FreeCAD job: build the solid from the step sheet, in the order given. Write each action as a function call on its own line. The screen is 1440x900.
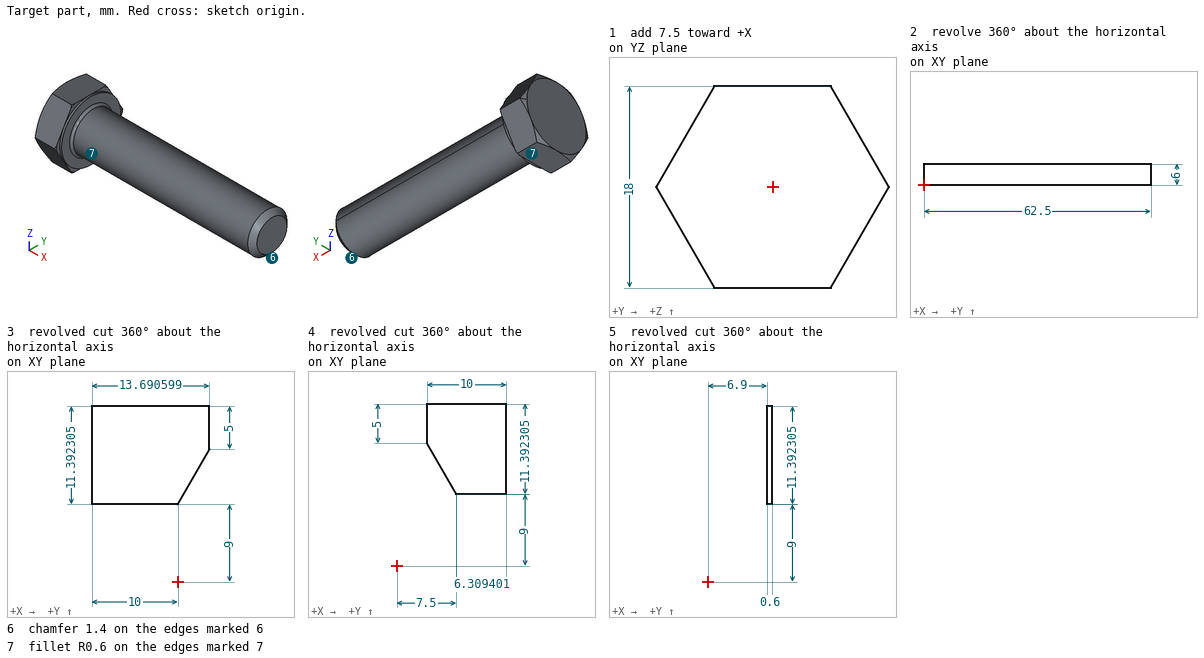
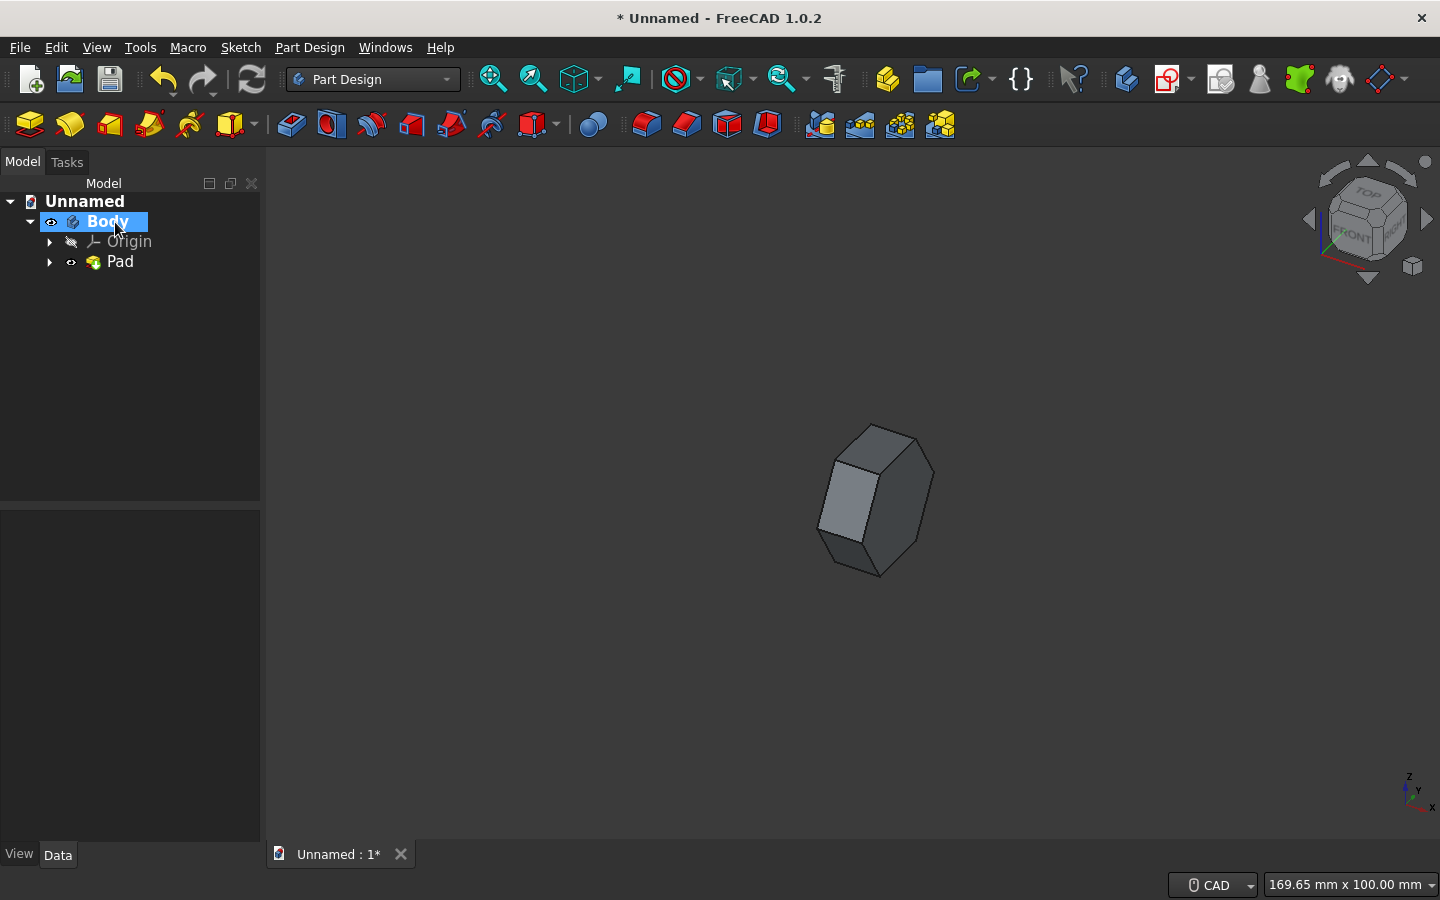
click(494, 80)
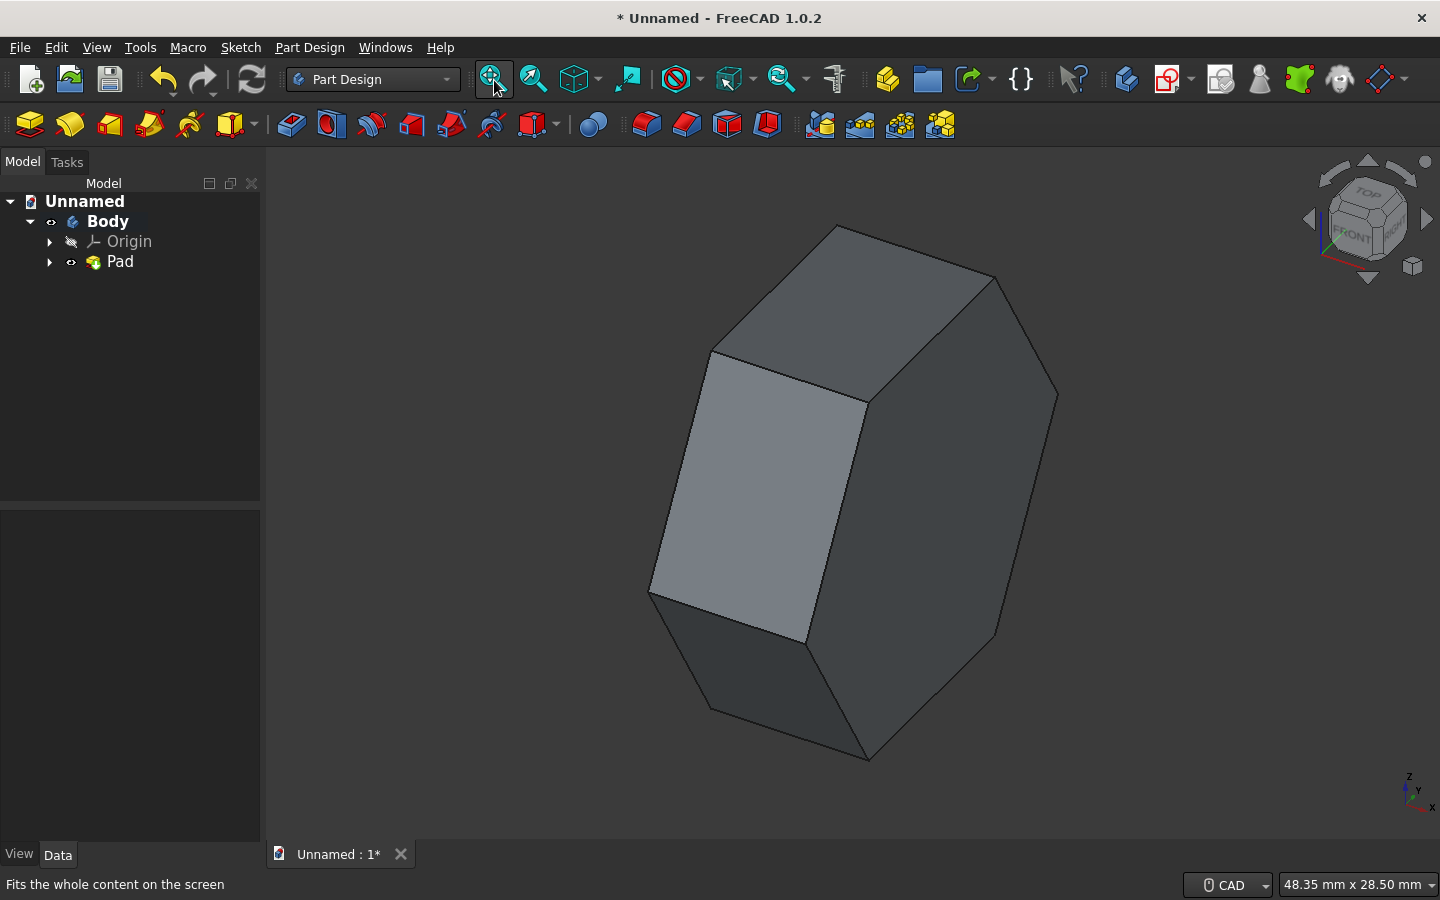
click(1168, 80)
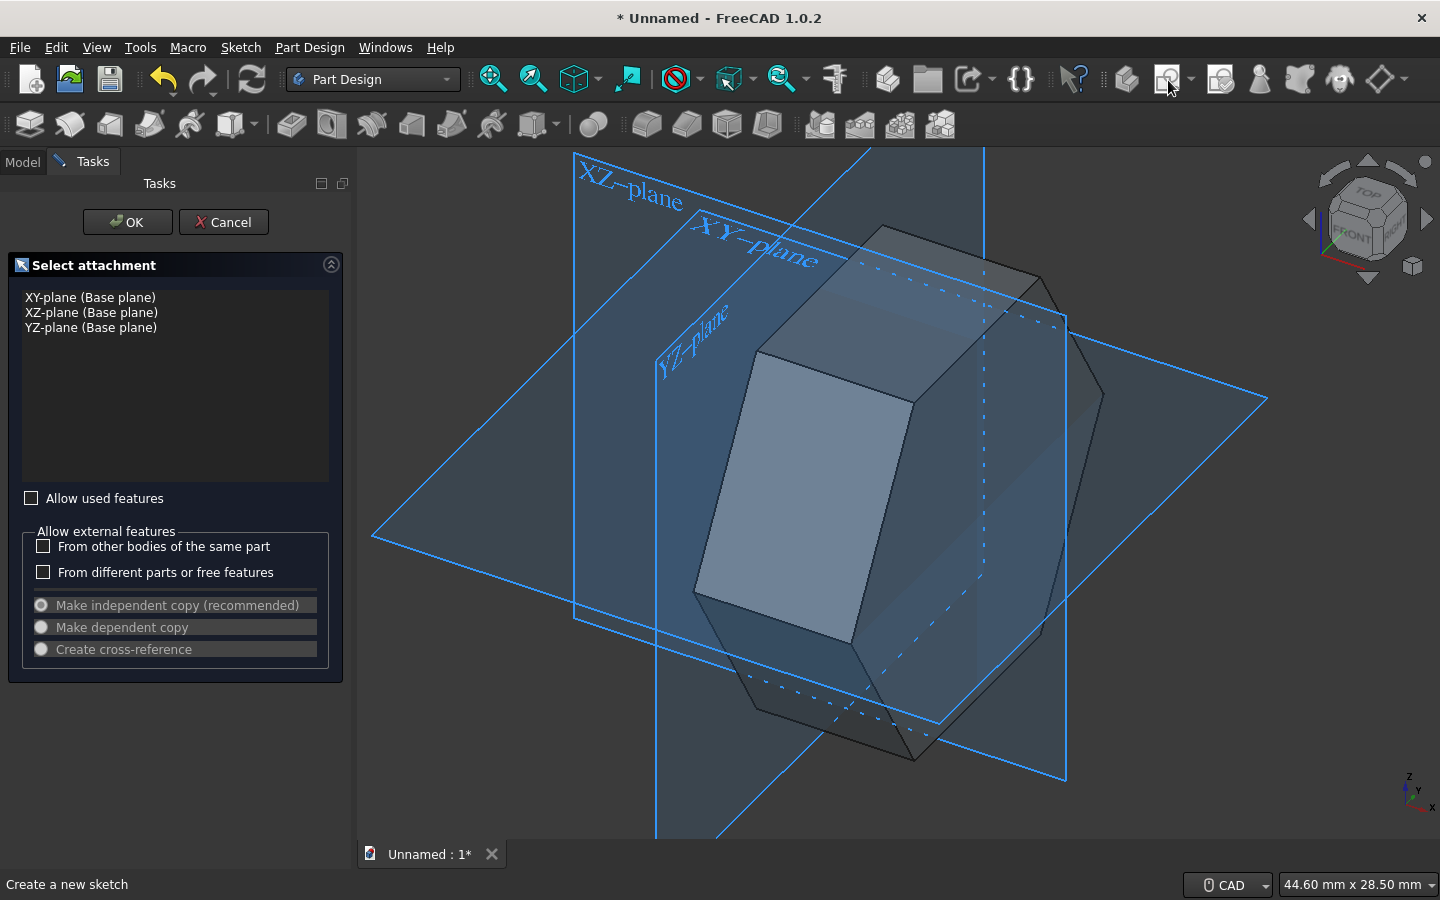
click(82, 298)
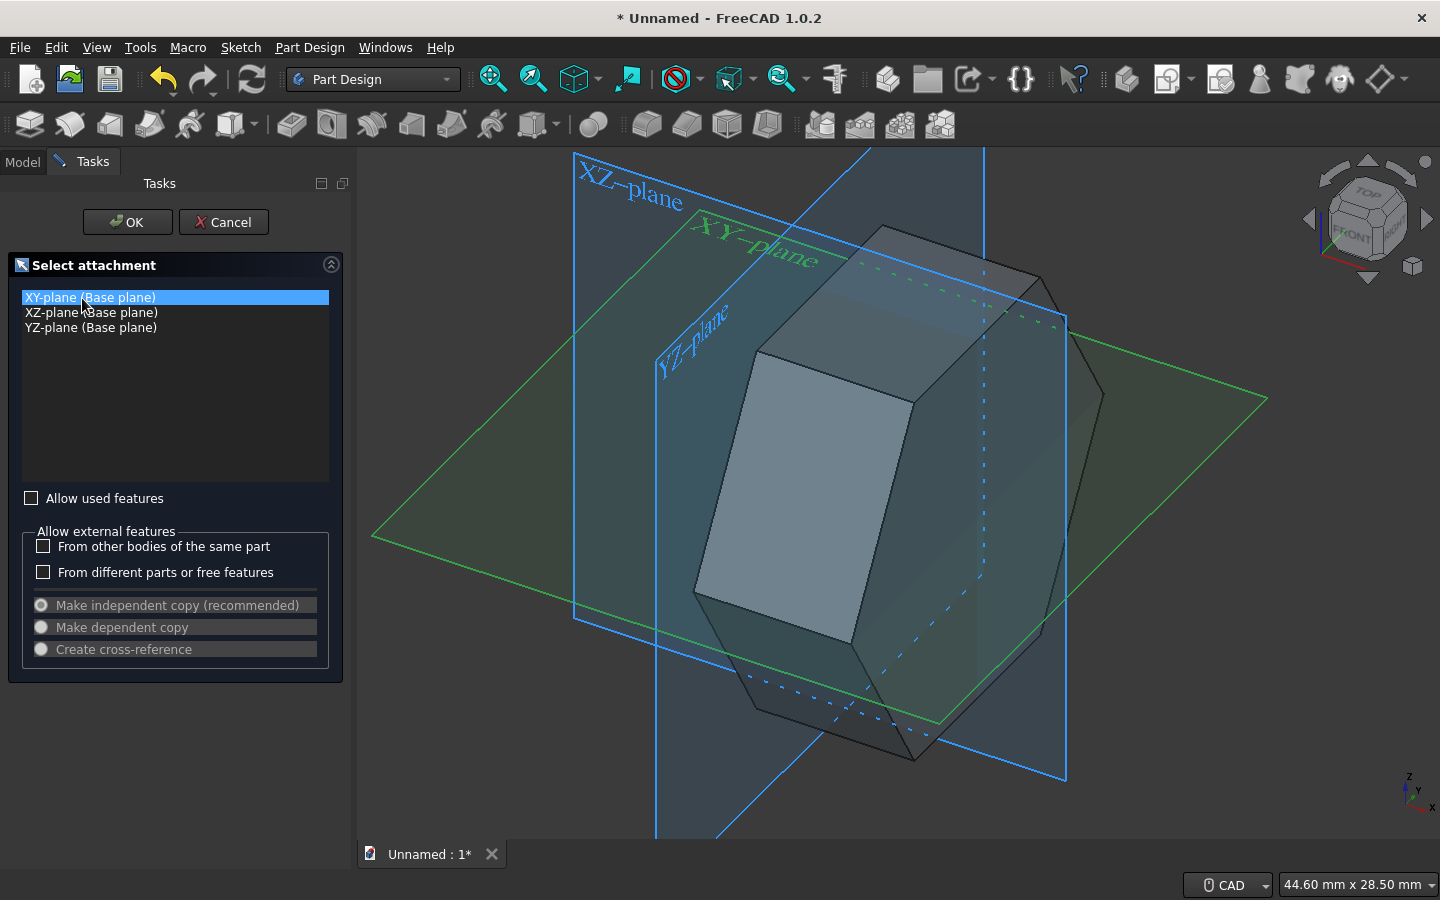
click(128, 222)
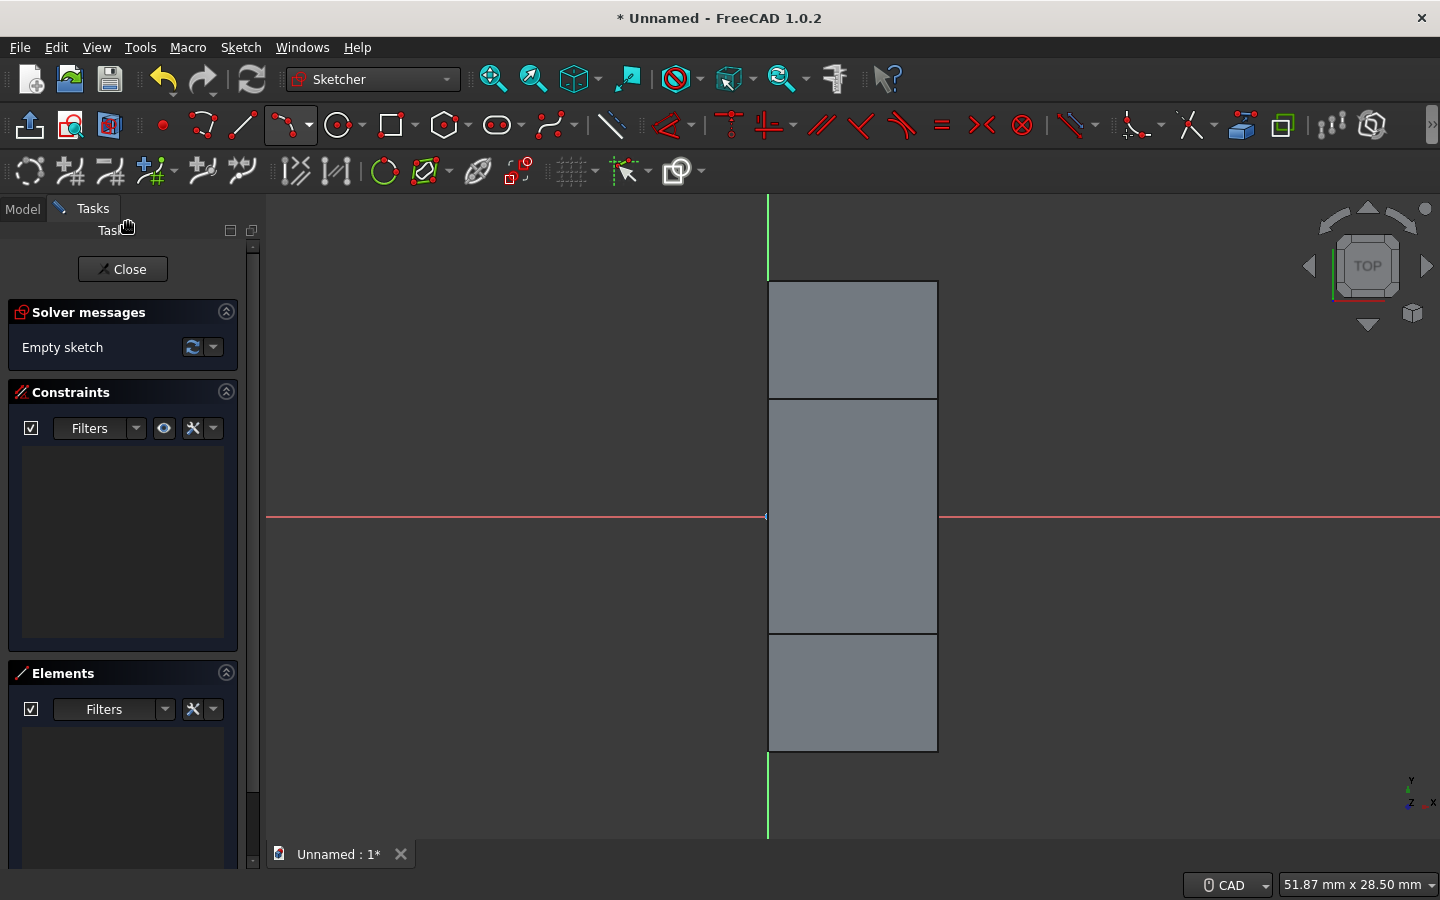
click(110, 126)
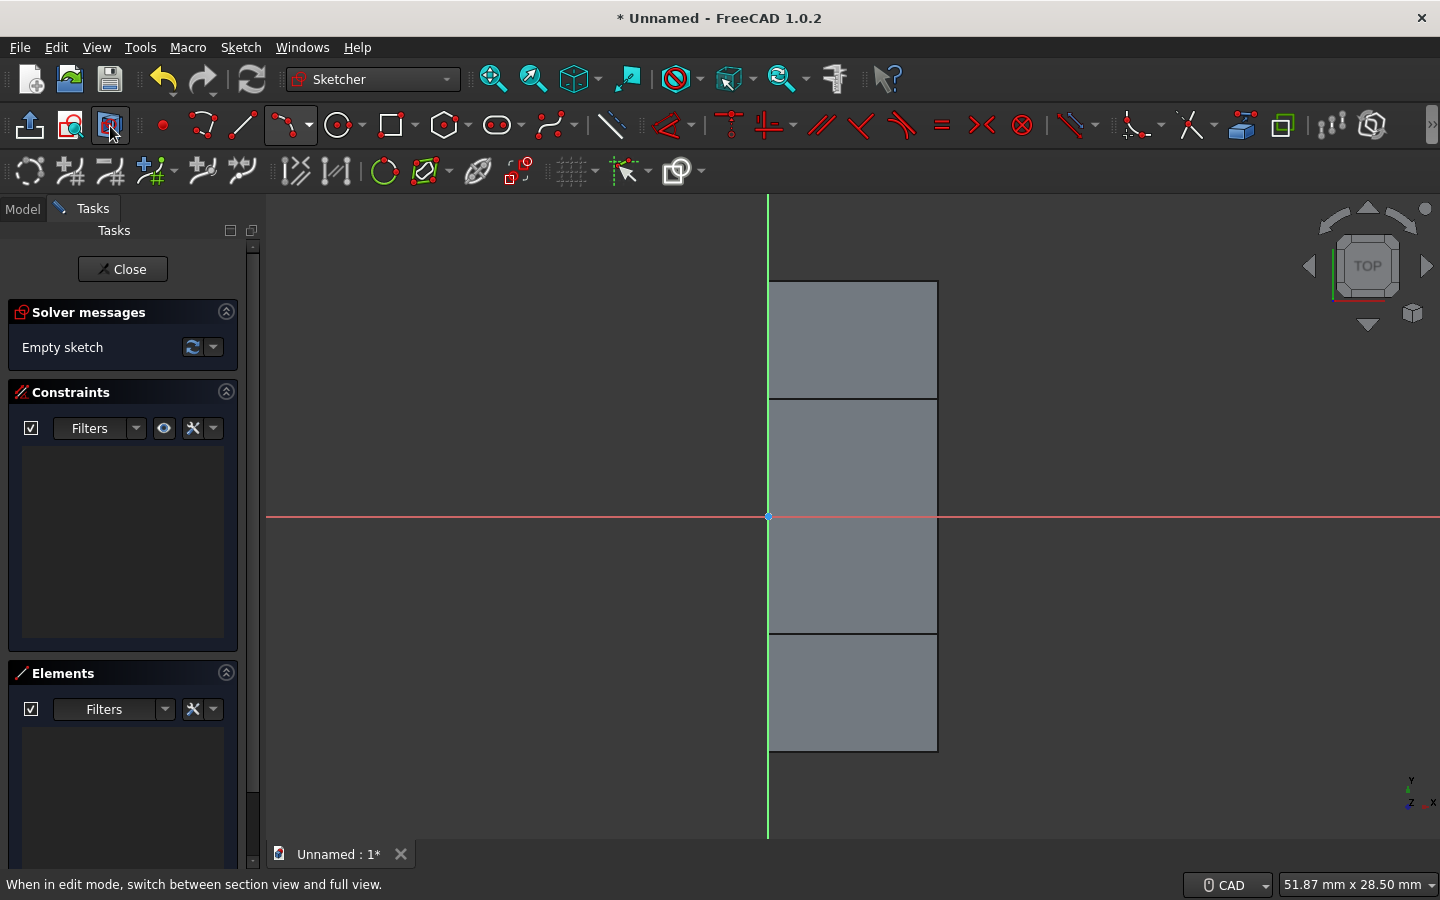
scroll(294, 572, down, 4)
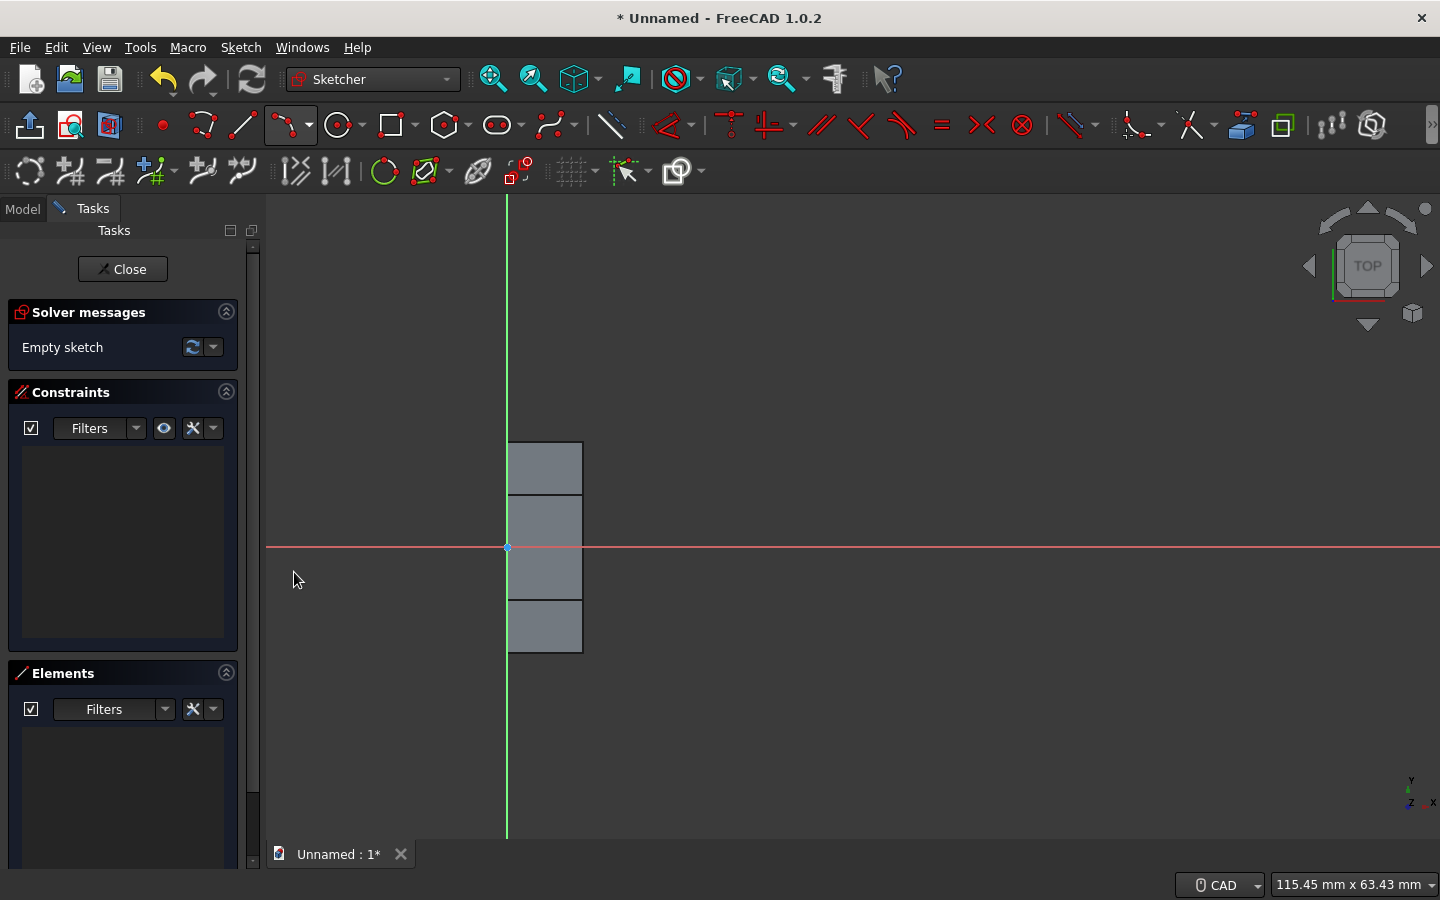
key(g)
key(r)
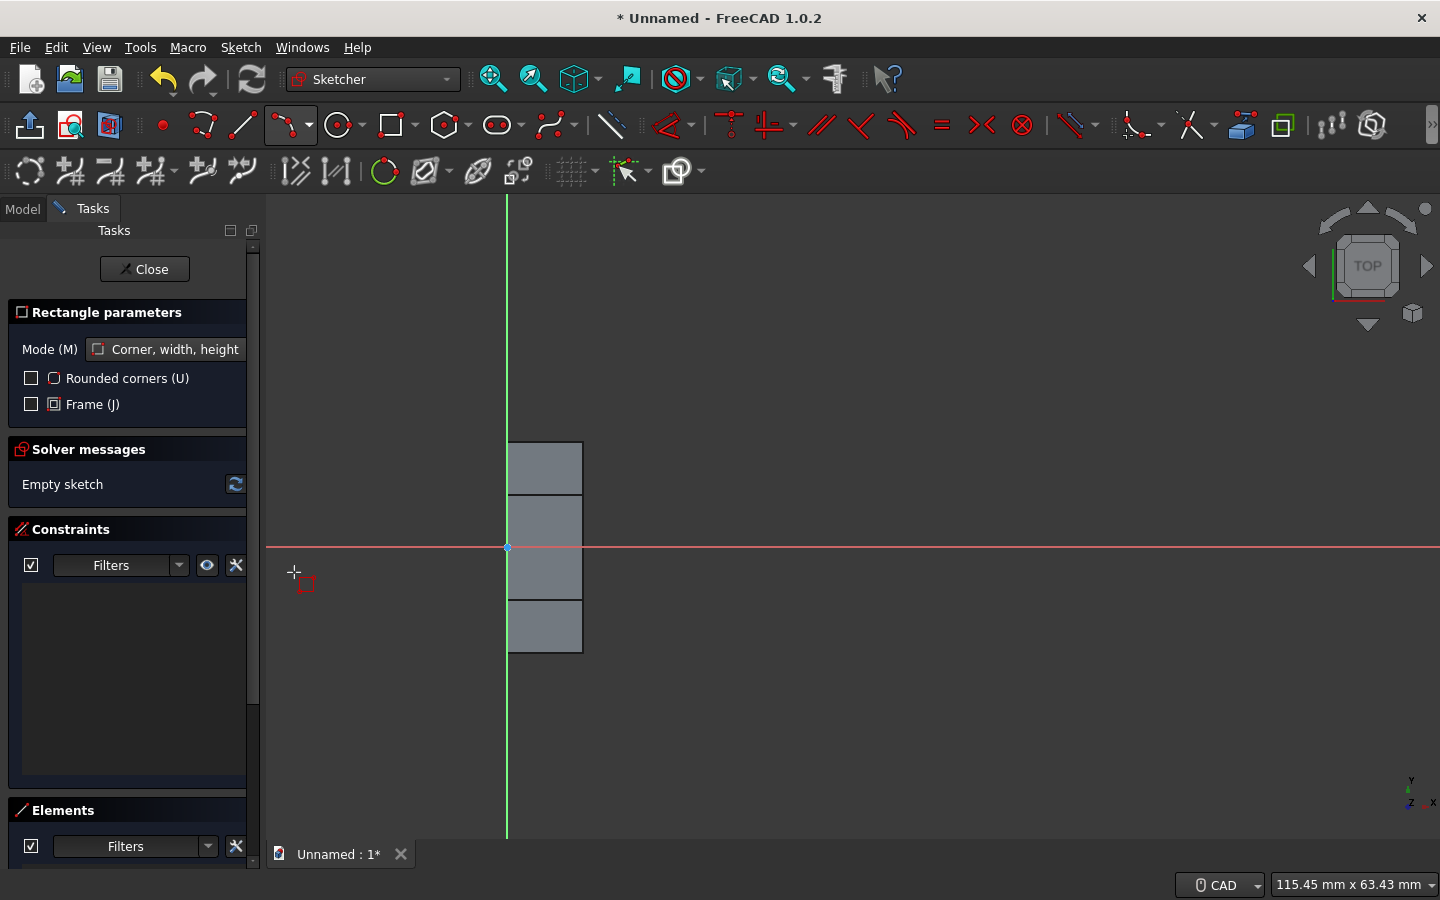
click(507, 547)
click(1143, 486)
key(Escape)